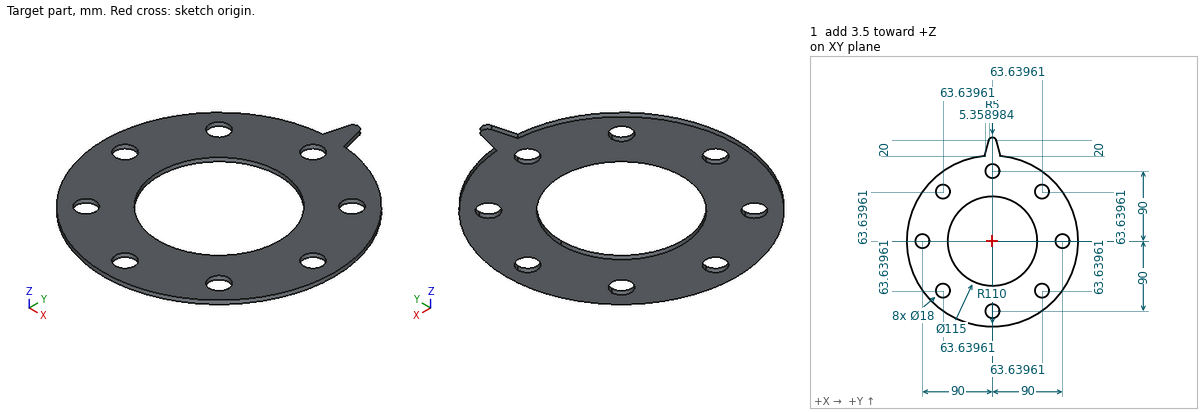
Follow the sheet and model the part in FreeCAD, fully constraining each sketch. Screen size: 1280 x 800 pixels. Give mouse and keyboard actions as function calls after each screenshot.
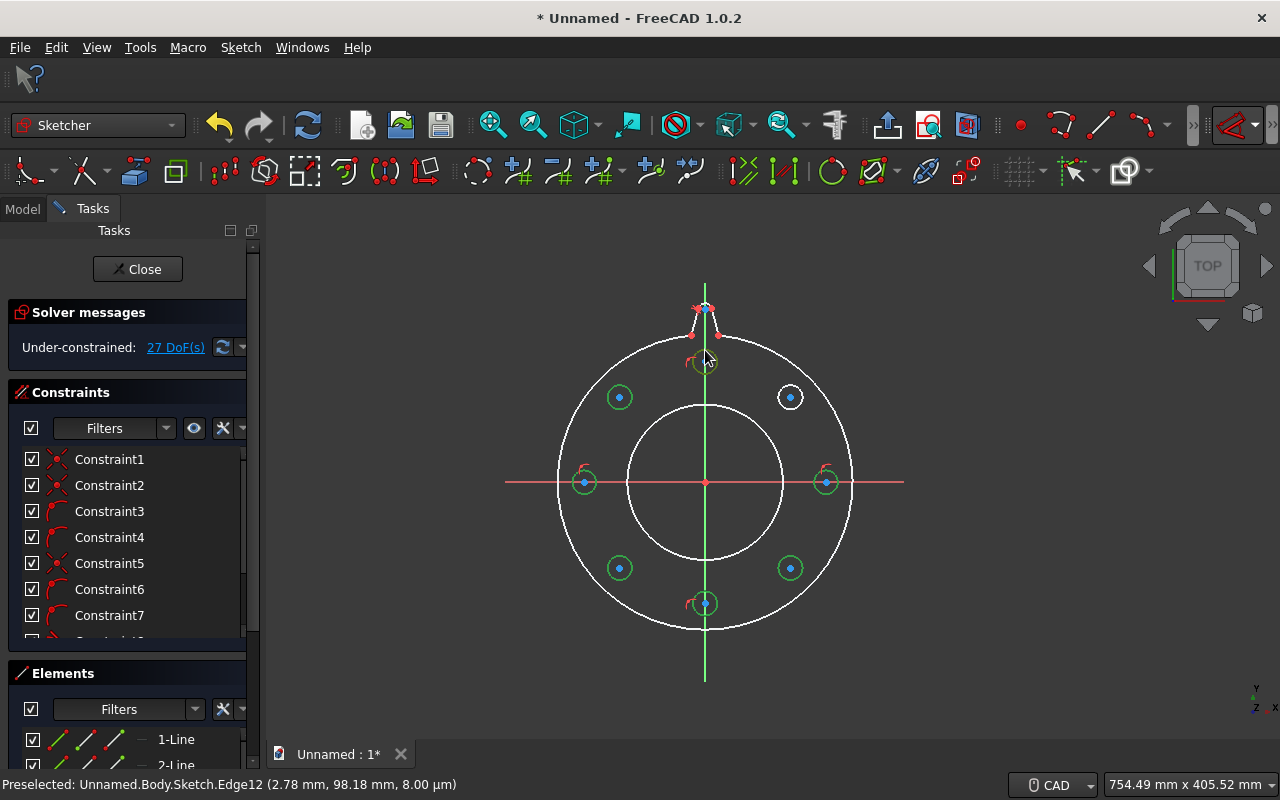
click(799, 389)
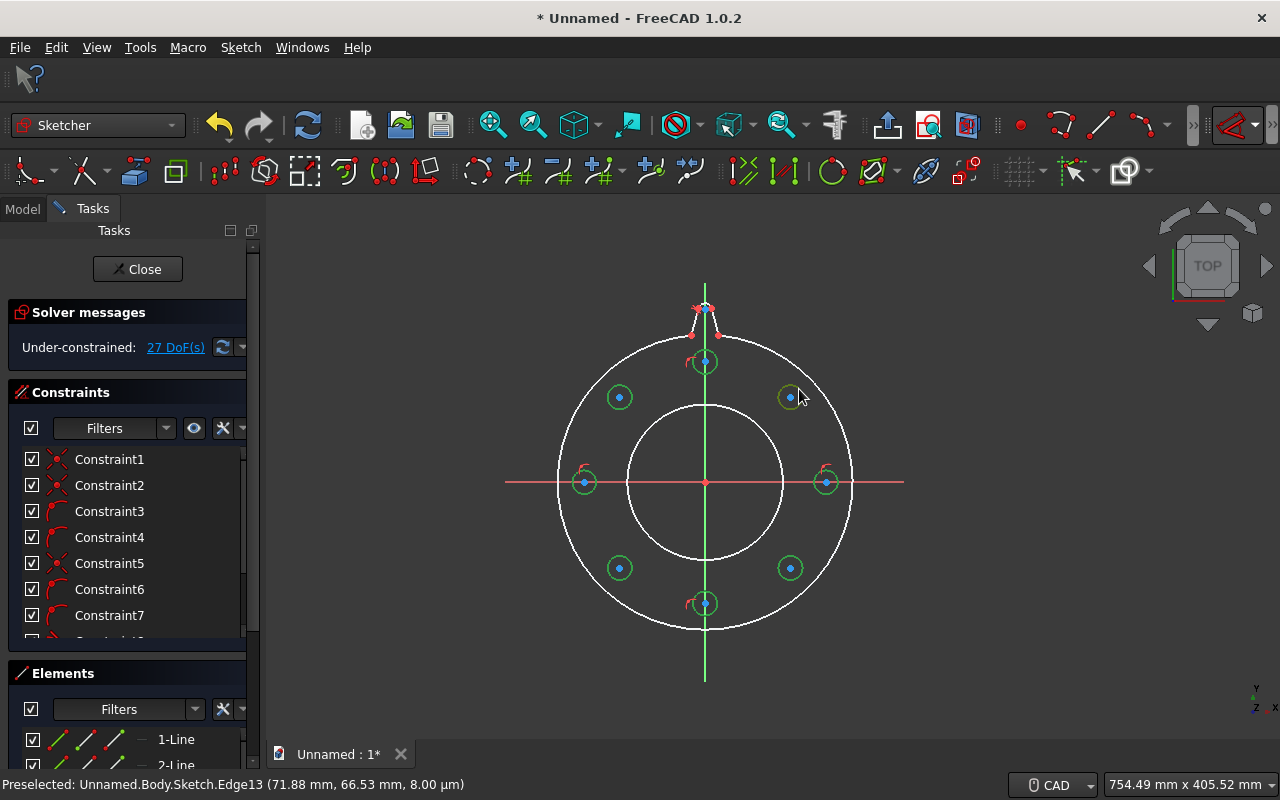
key(e)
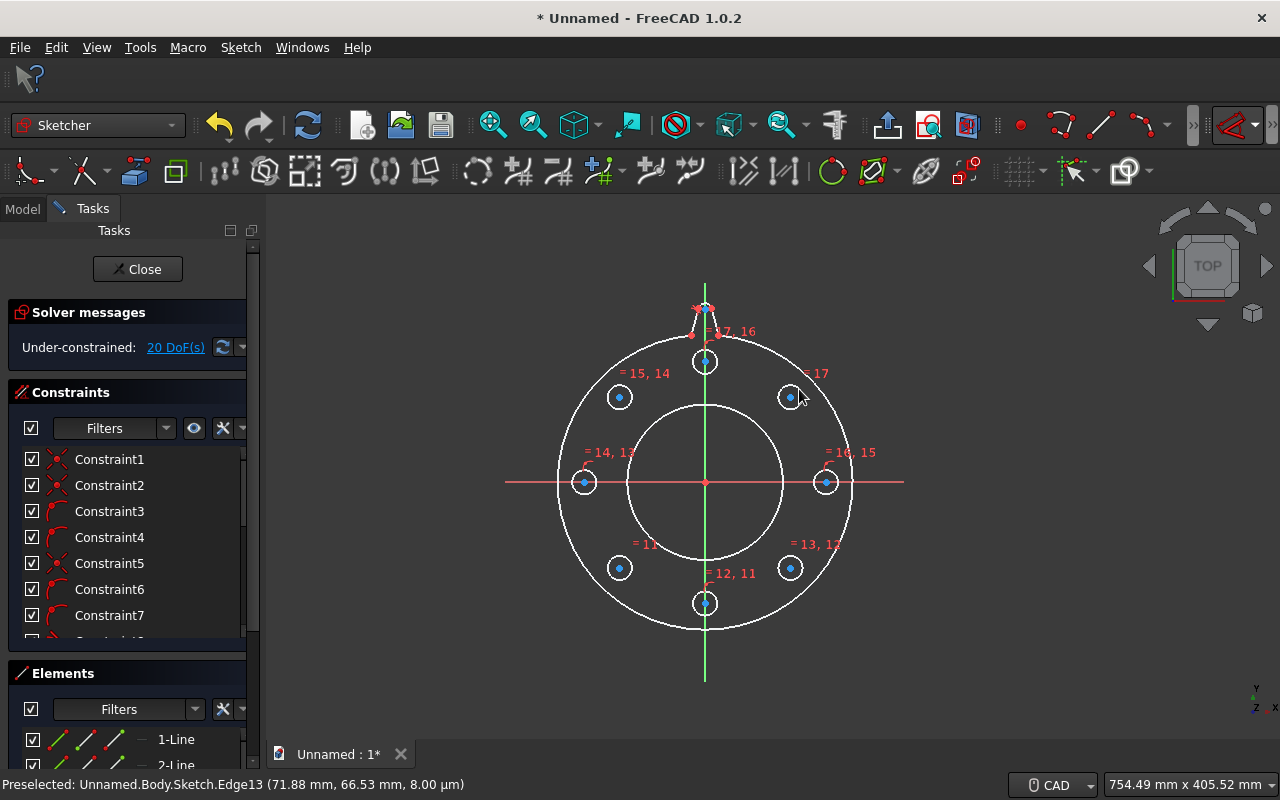
scroll(705, 310, up, 4)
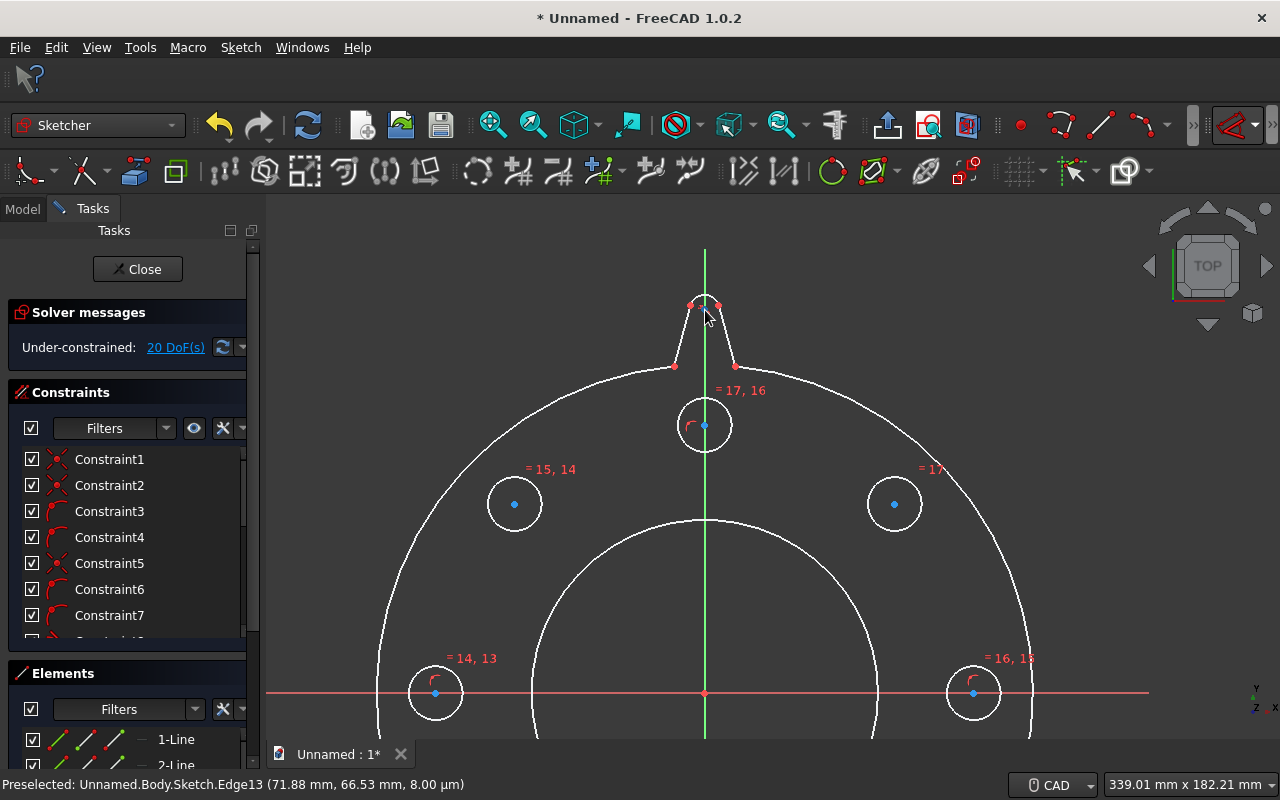
click(705, 310)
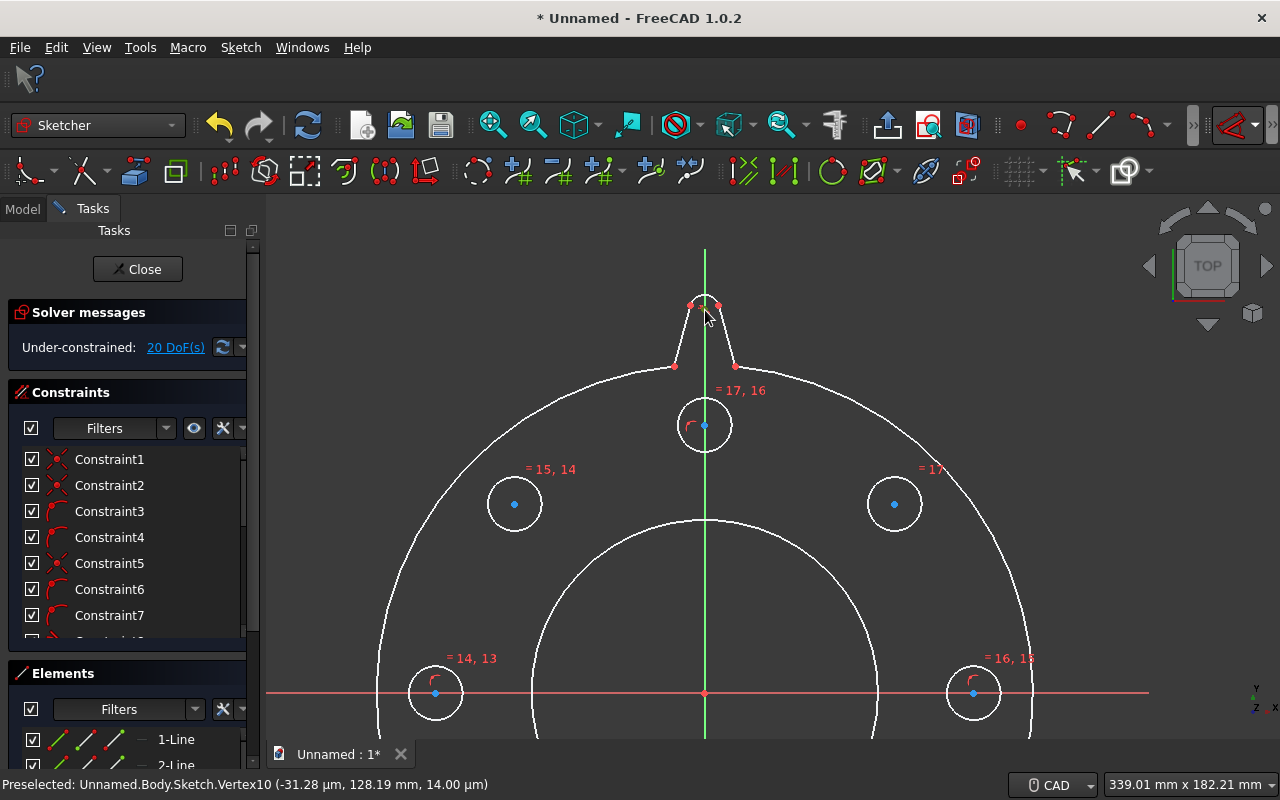
click(705, 641)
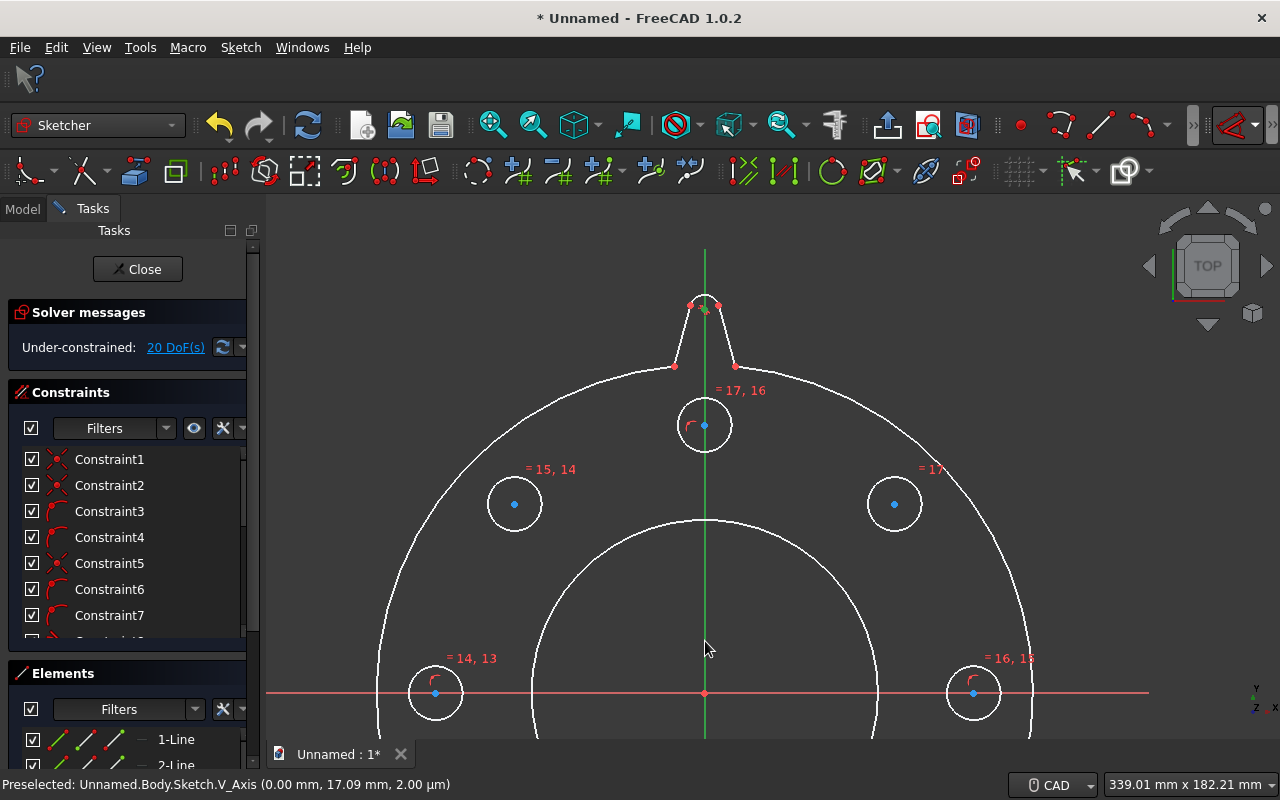
key(c)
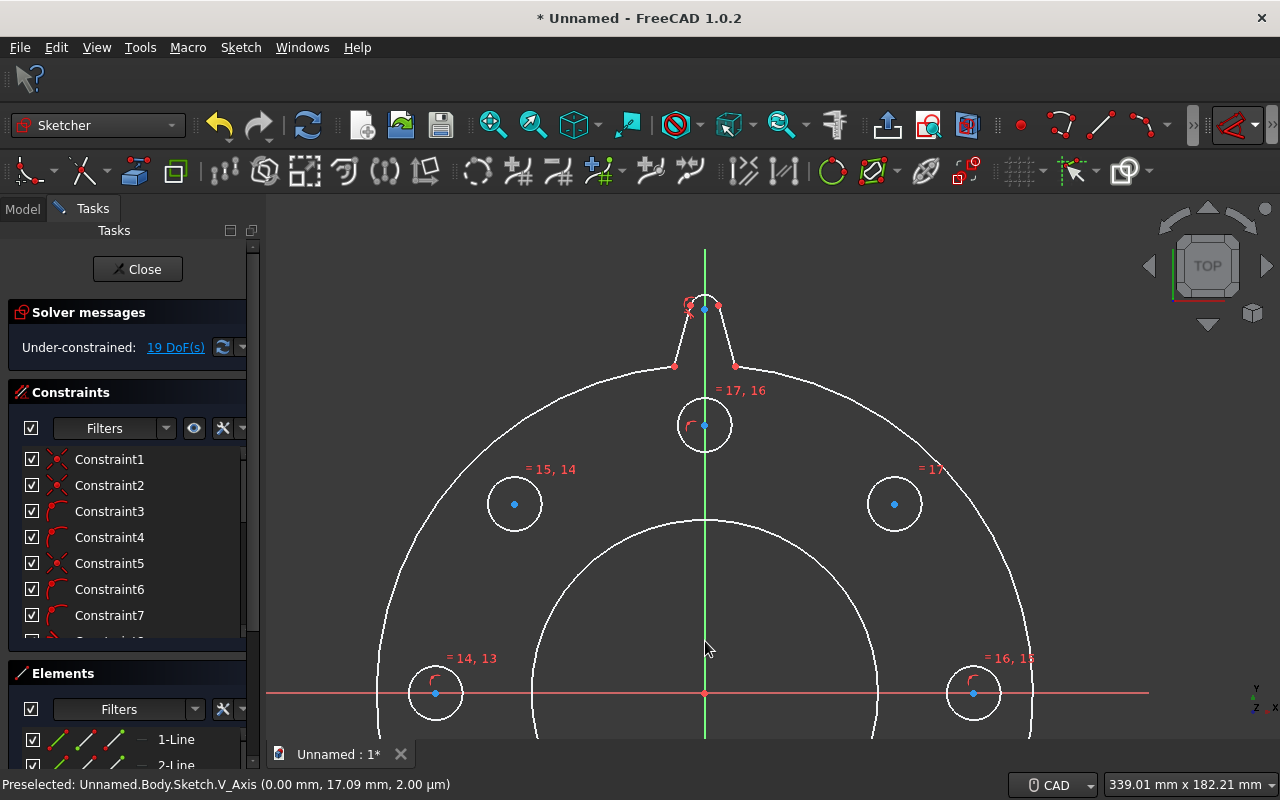
click(1232, 126)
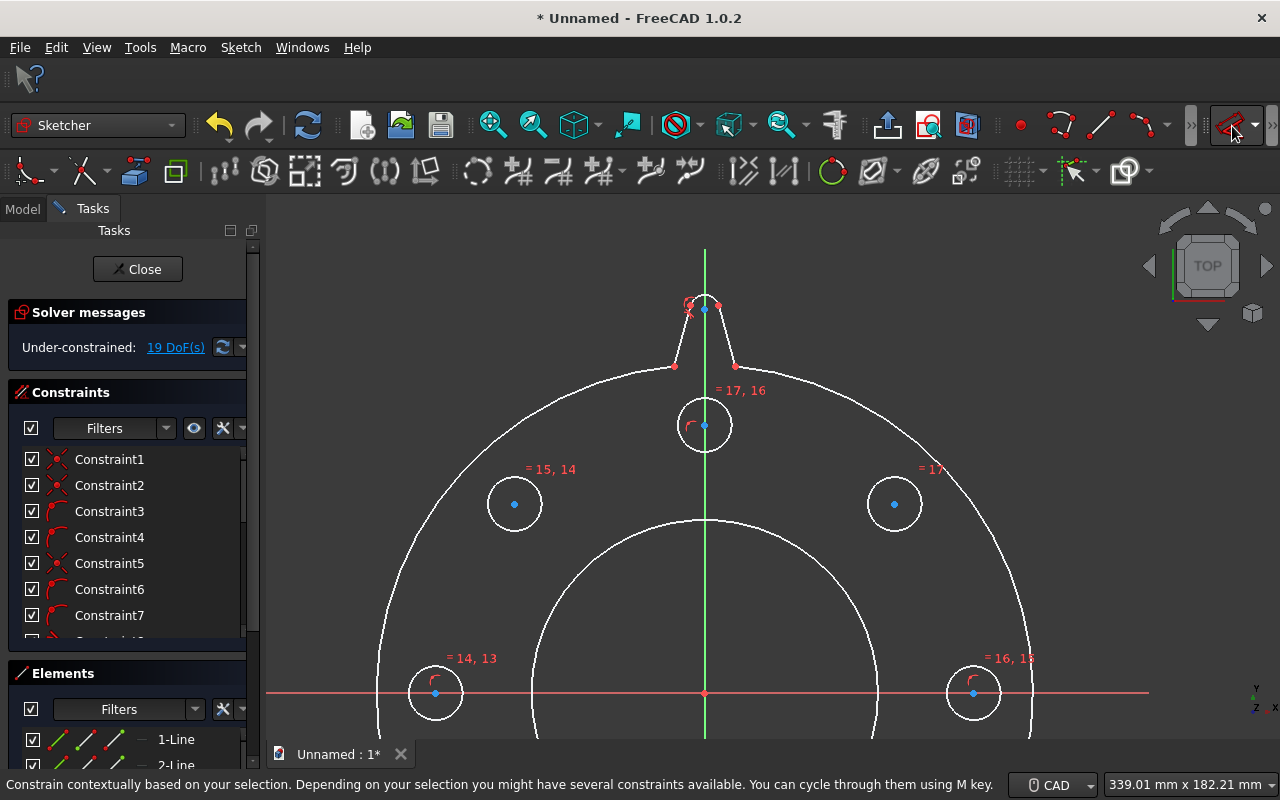
click(387, 609)
click(356, 601)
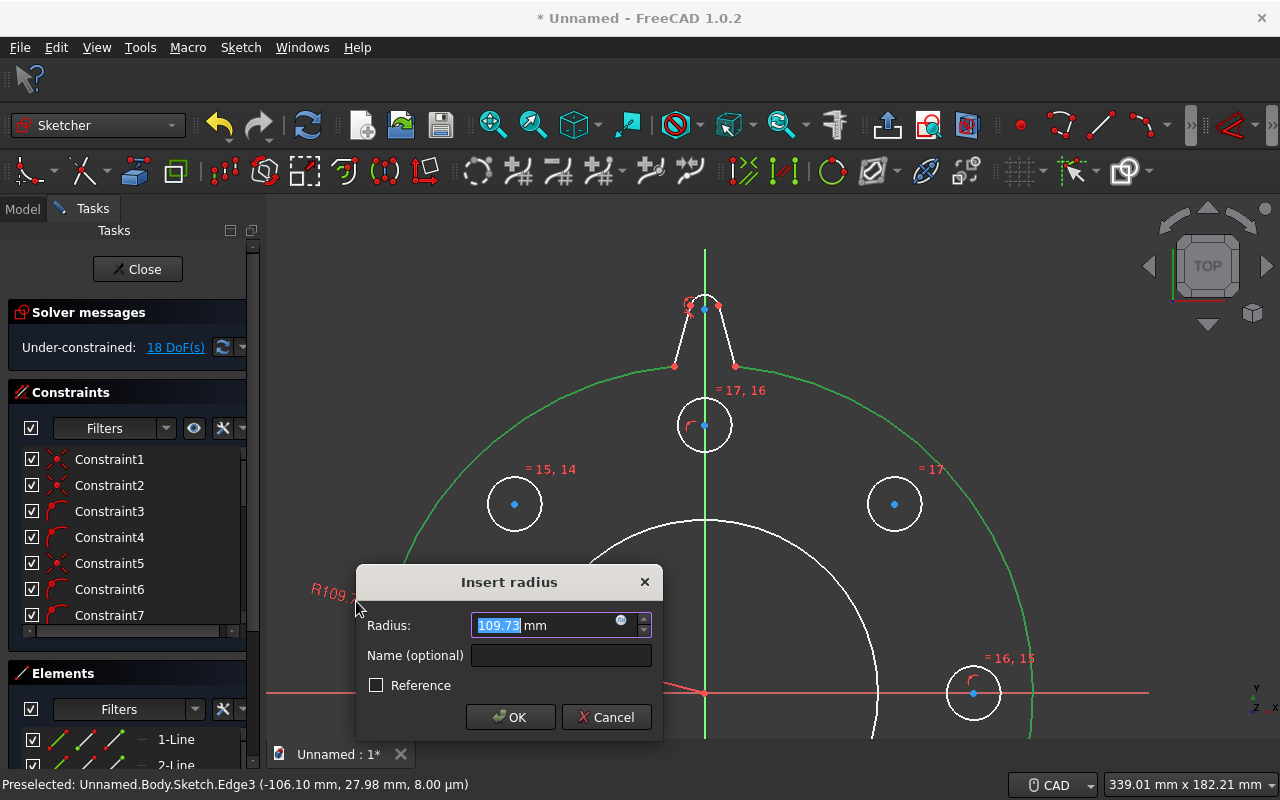
text(110)
key(Return)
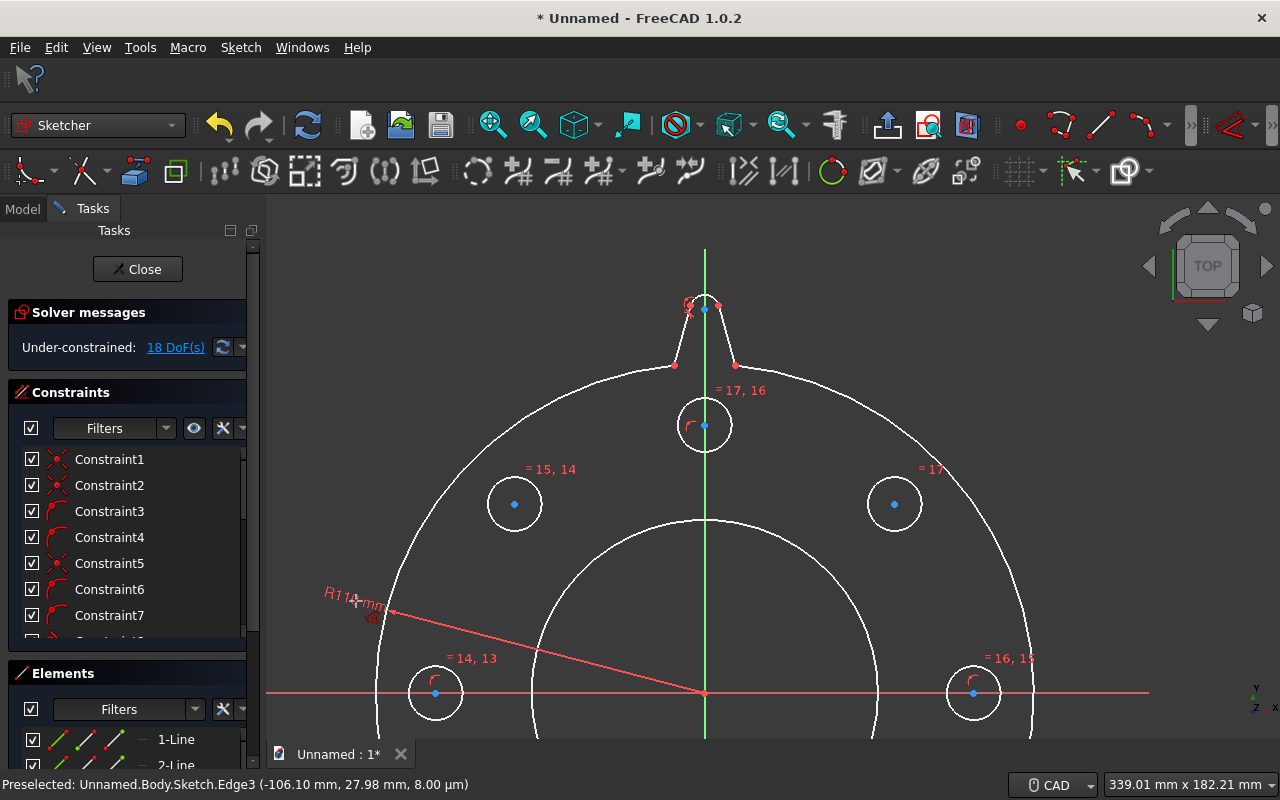
scroll(705, 295, up, 5)